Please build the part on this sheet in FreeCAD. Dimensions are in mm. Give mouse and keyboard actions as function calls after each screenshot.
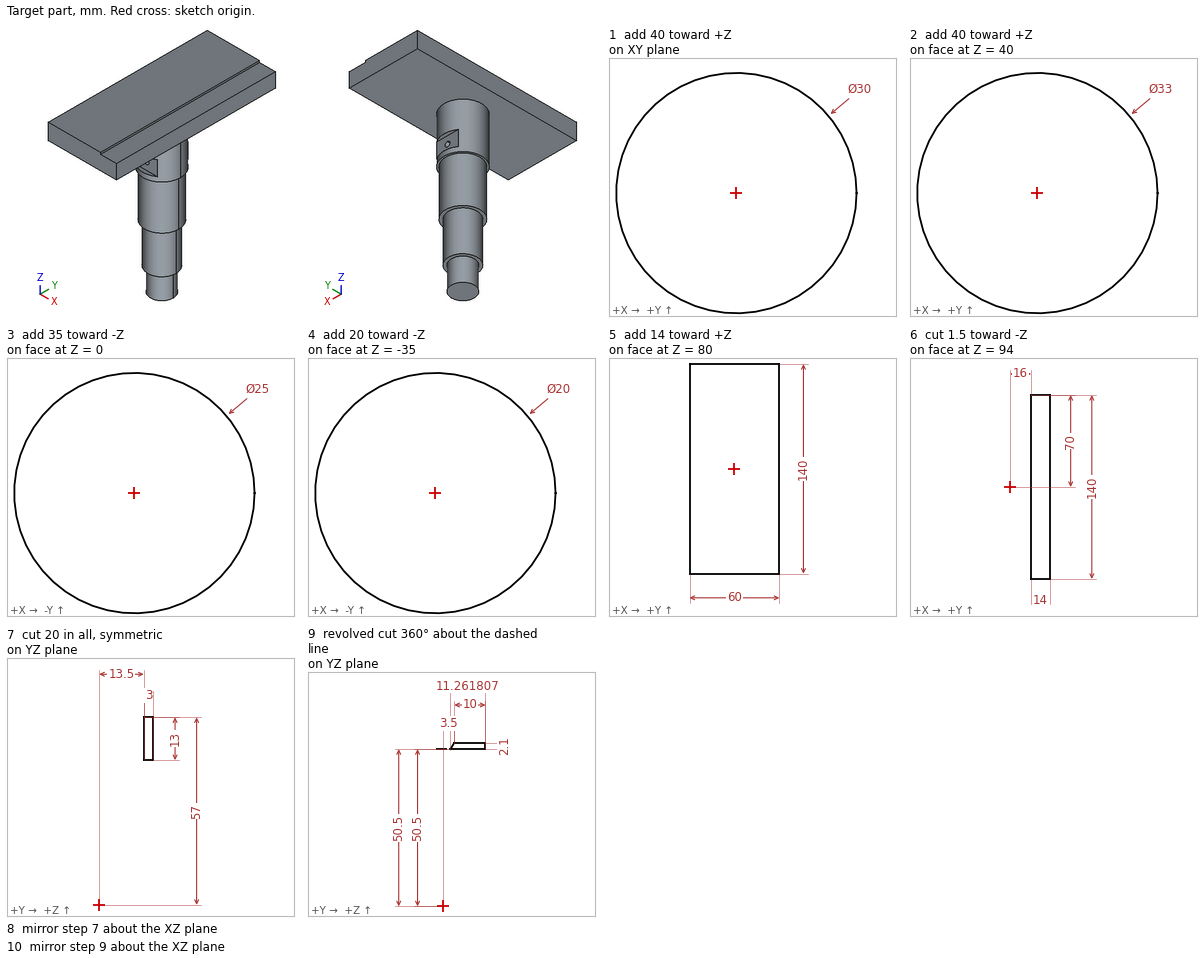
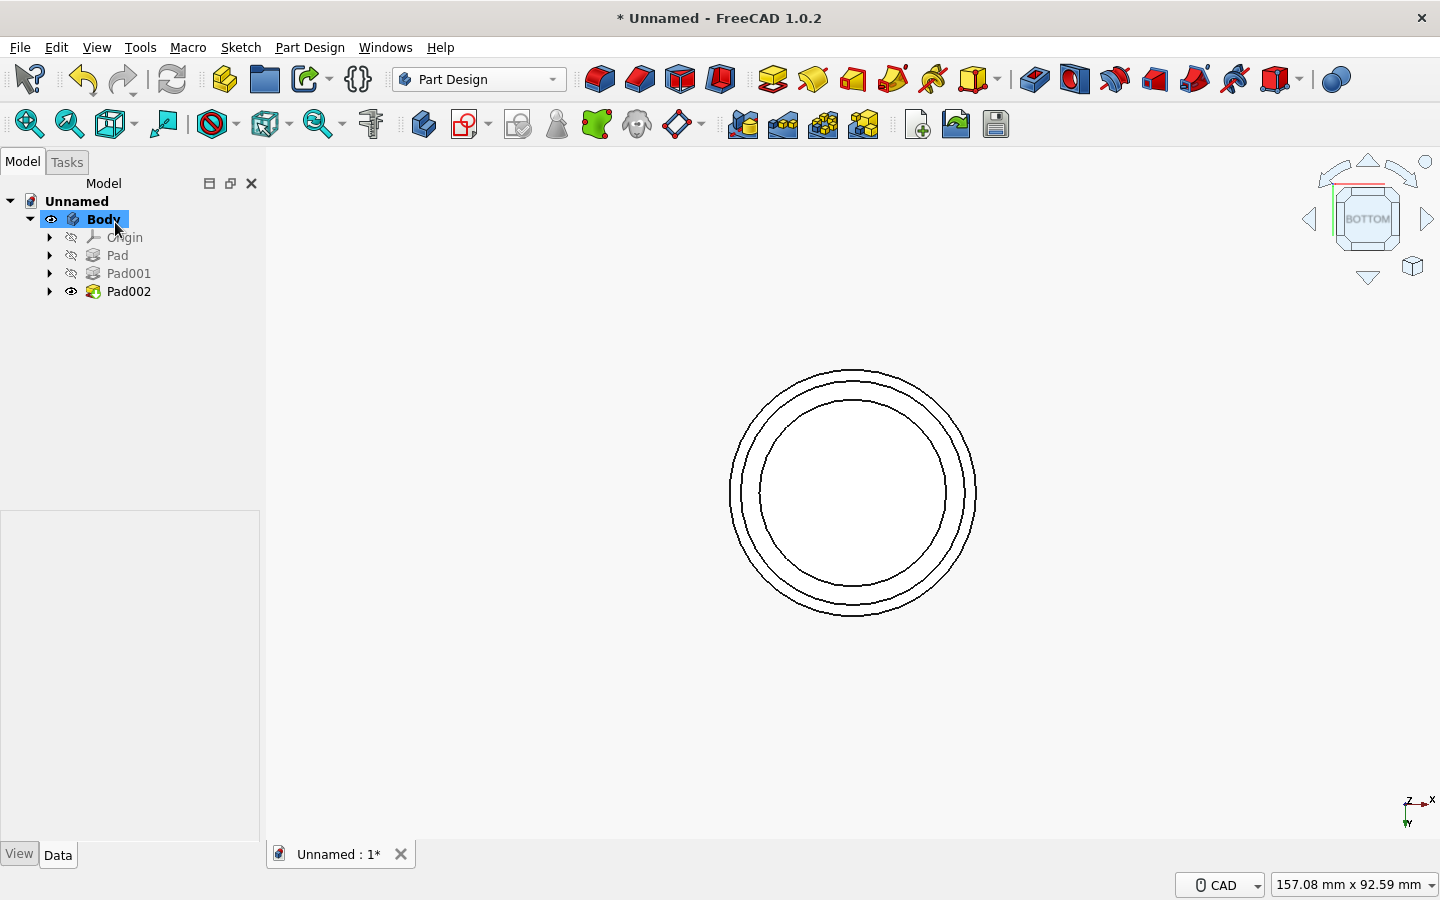
click(30, 124)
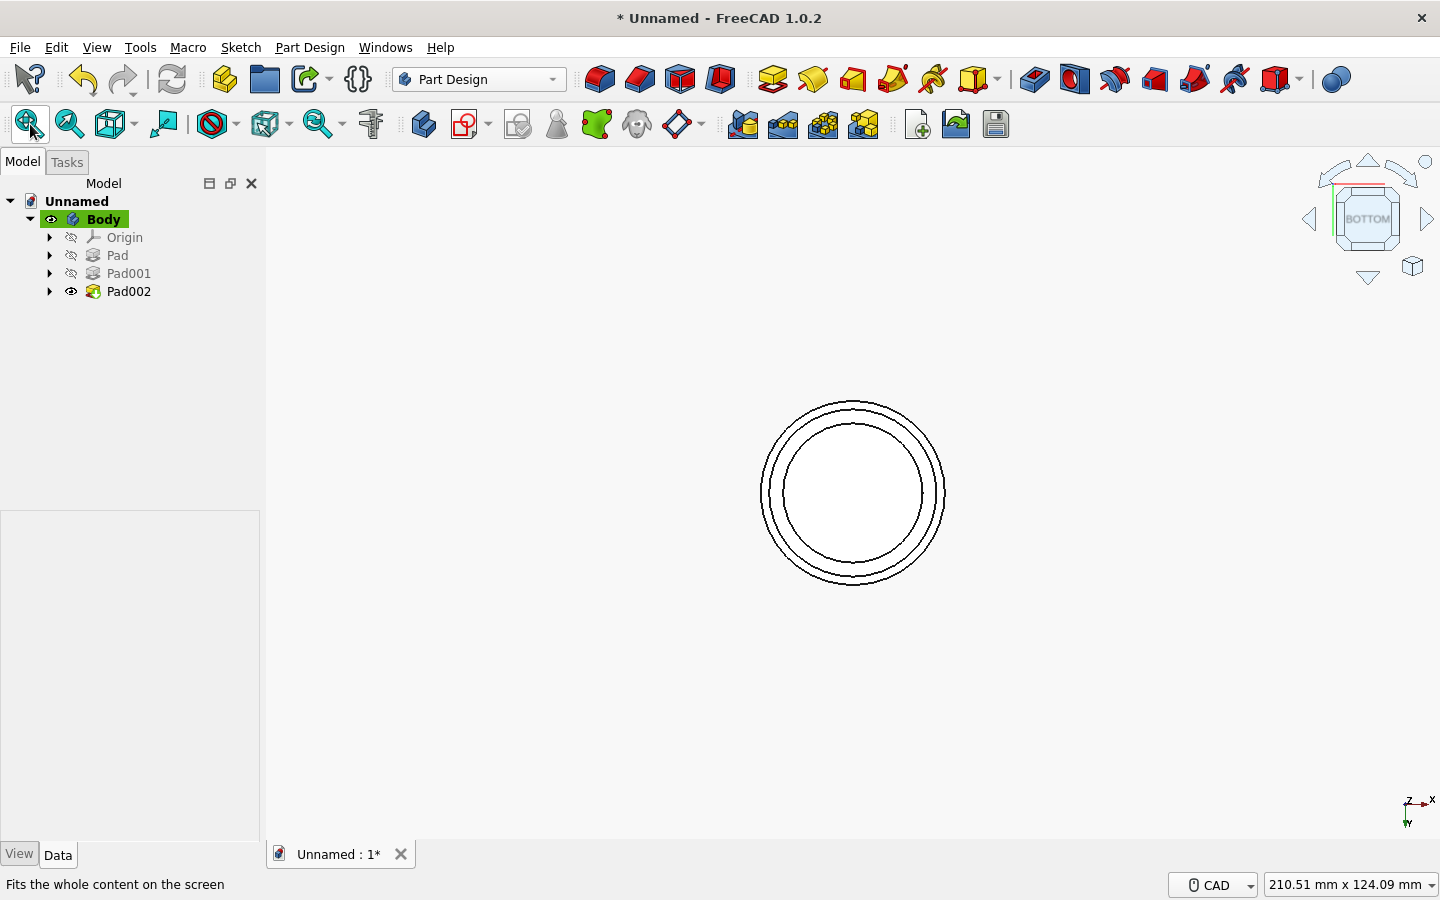
click(853, 492)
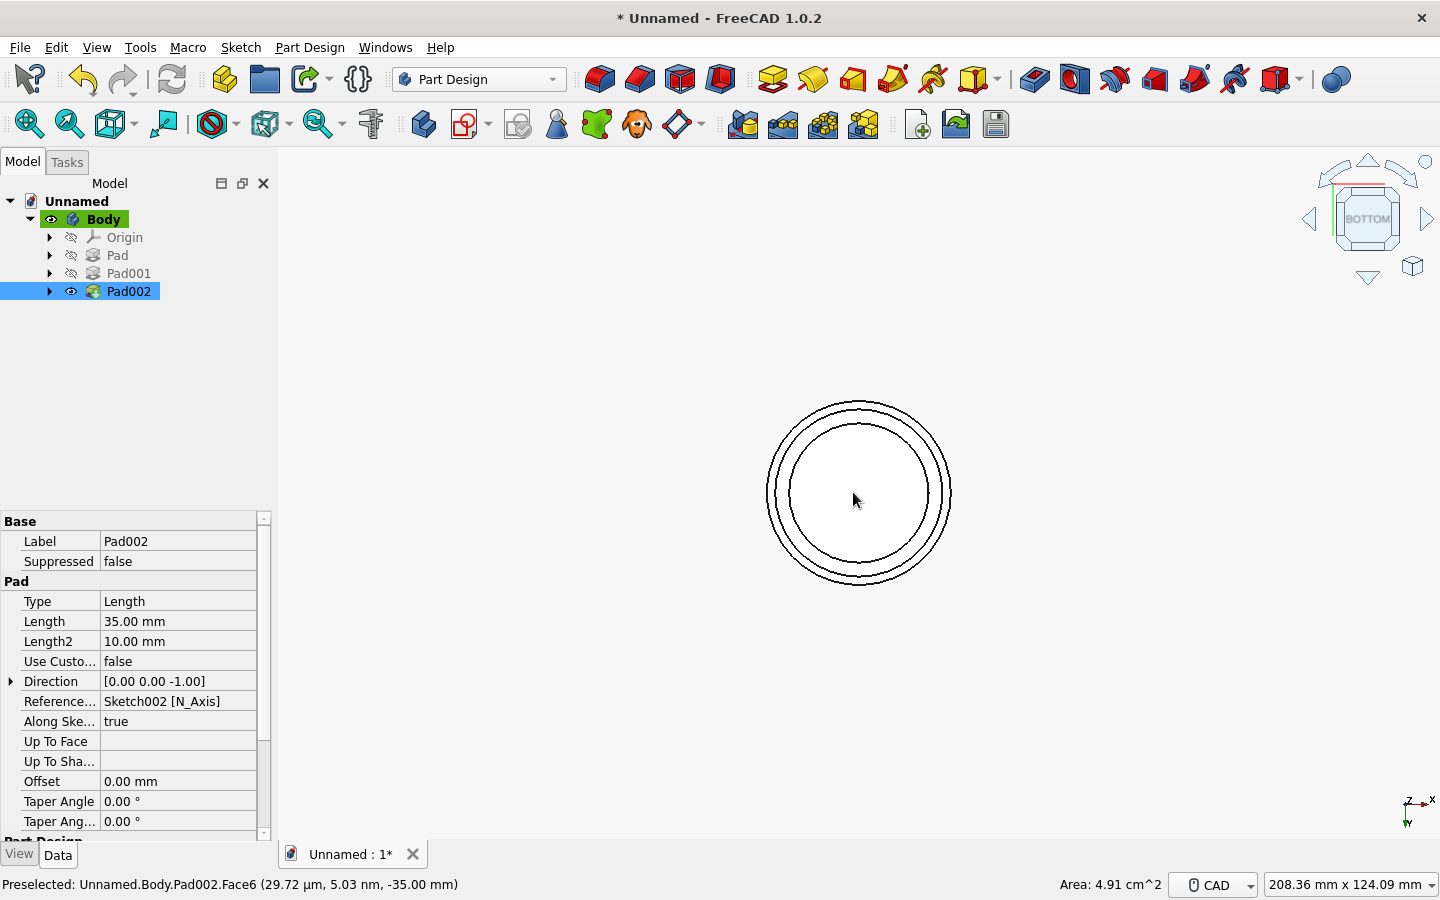
click(464, 124)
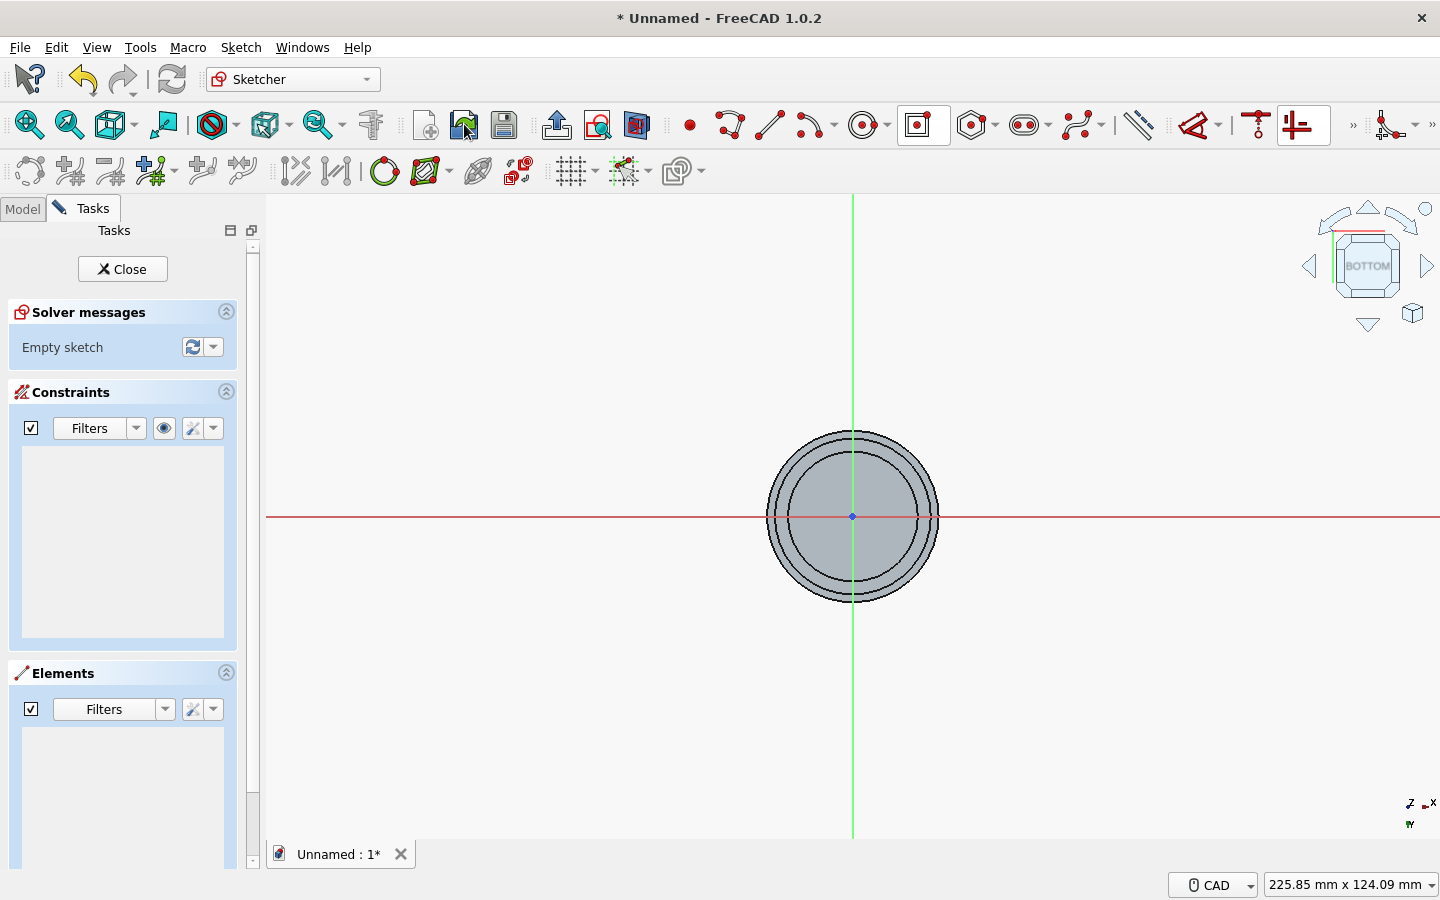
scroll(875, 516, up, 7)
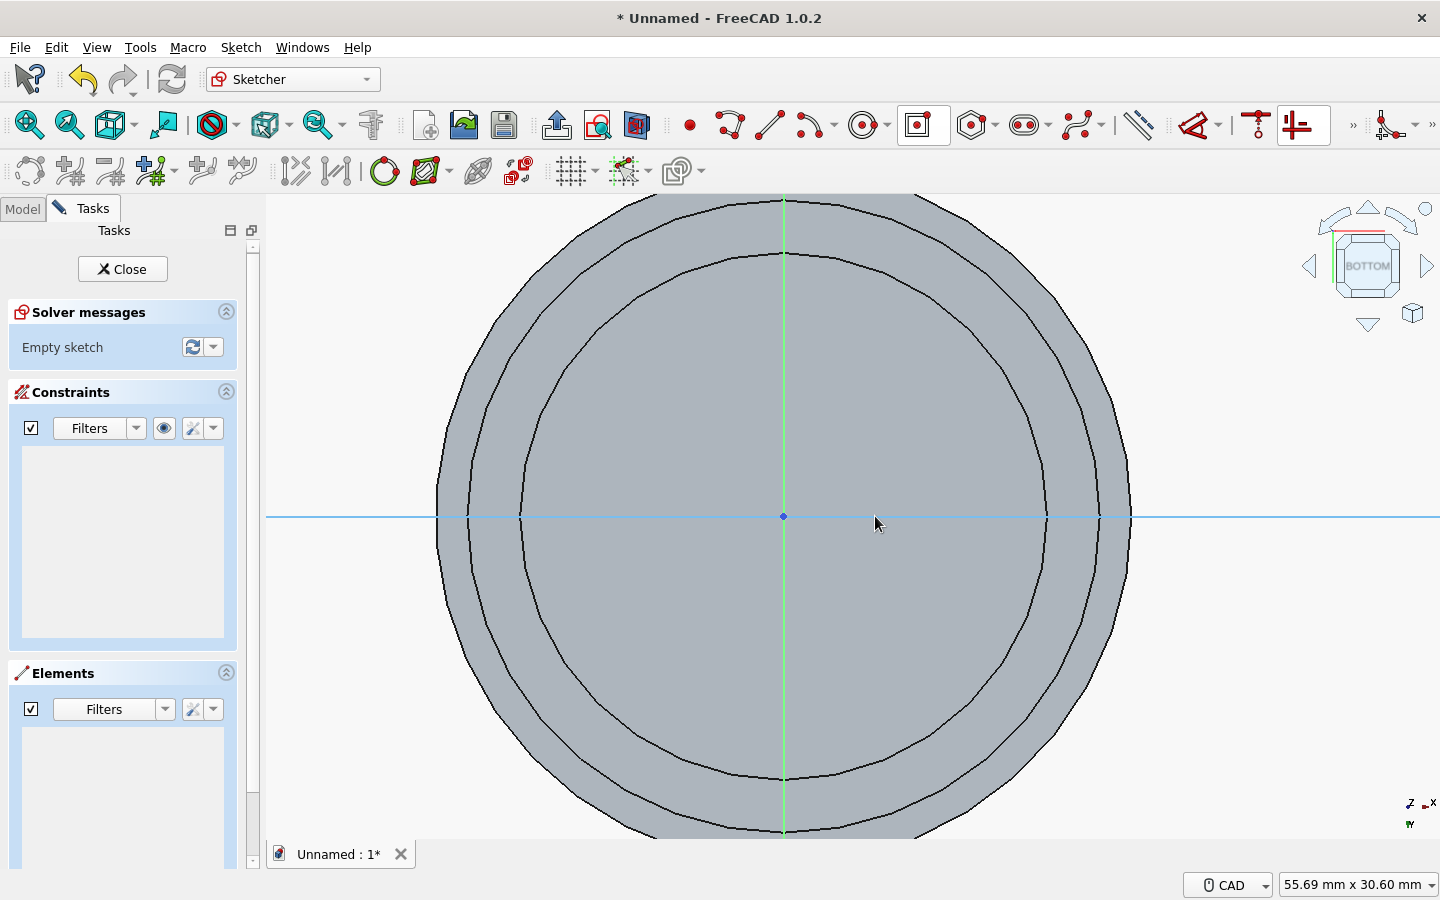
click(864, 126)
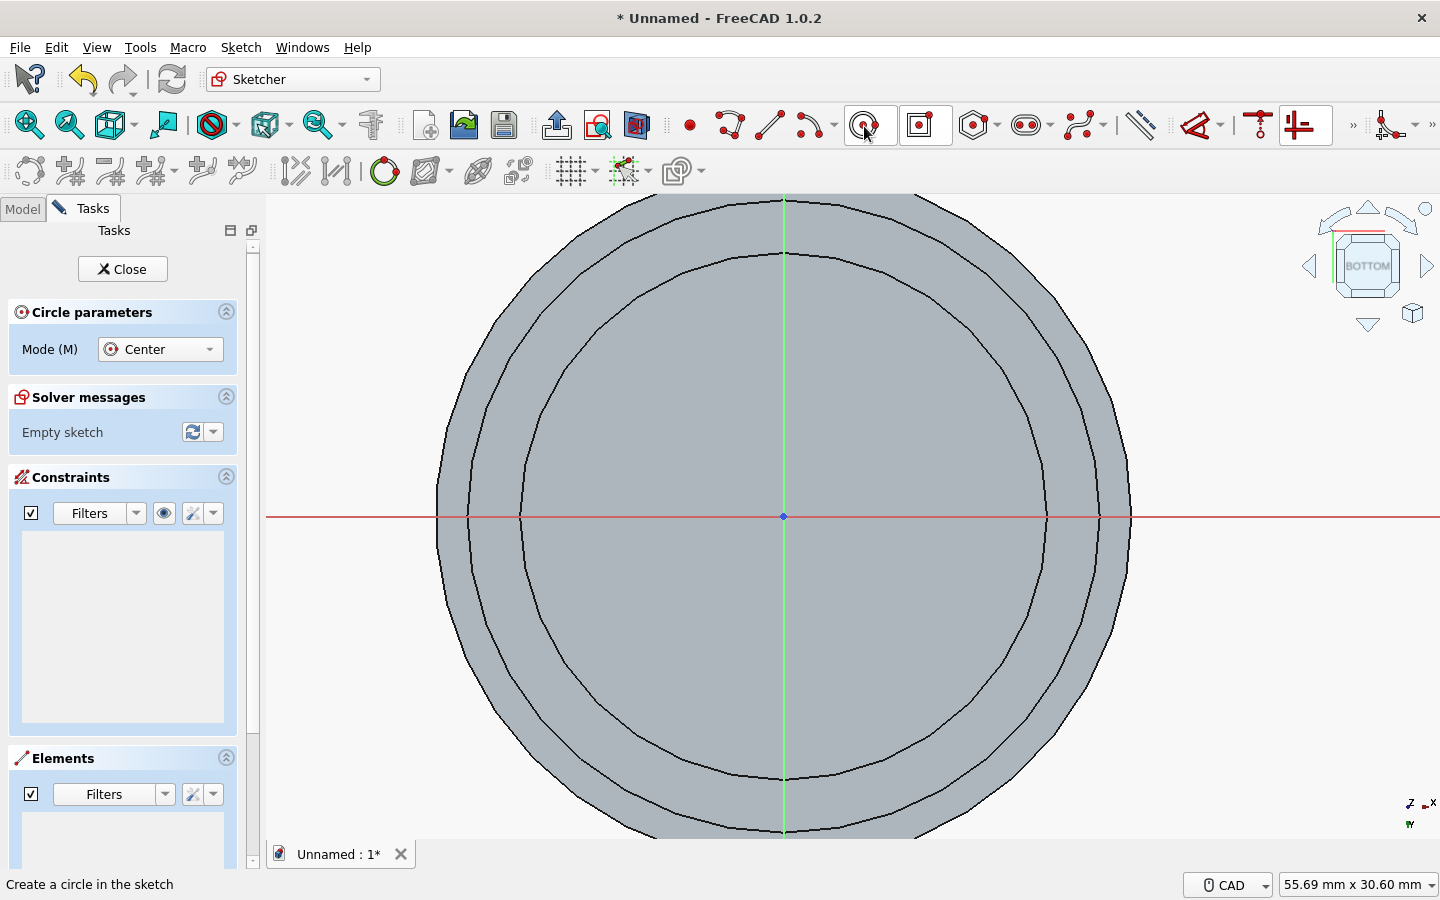
click(784, 516)
move(933, 367)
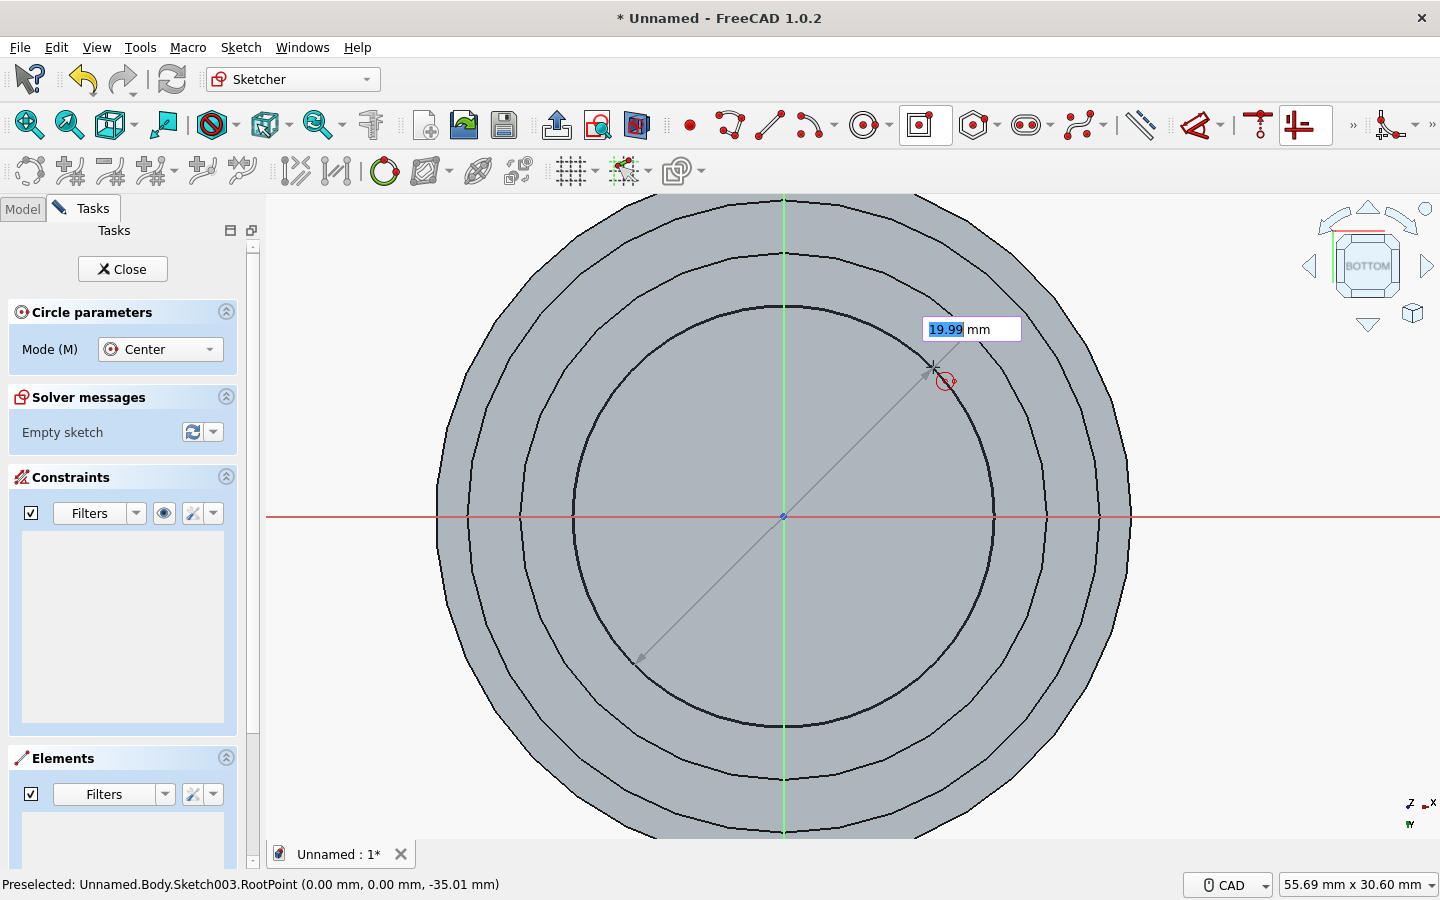
text(20)
key(Return)
key(Escape)